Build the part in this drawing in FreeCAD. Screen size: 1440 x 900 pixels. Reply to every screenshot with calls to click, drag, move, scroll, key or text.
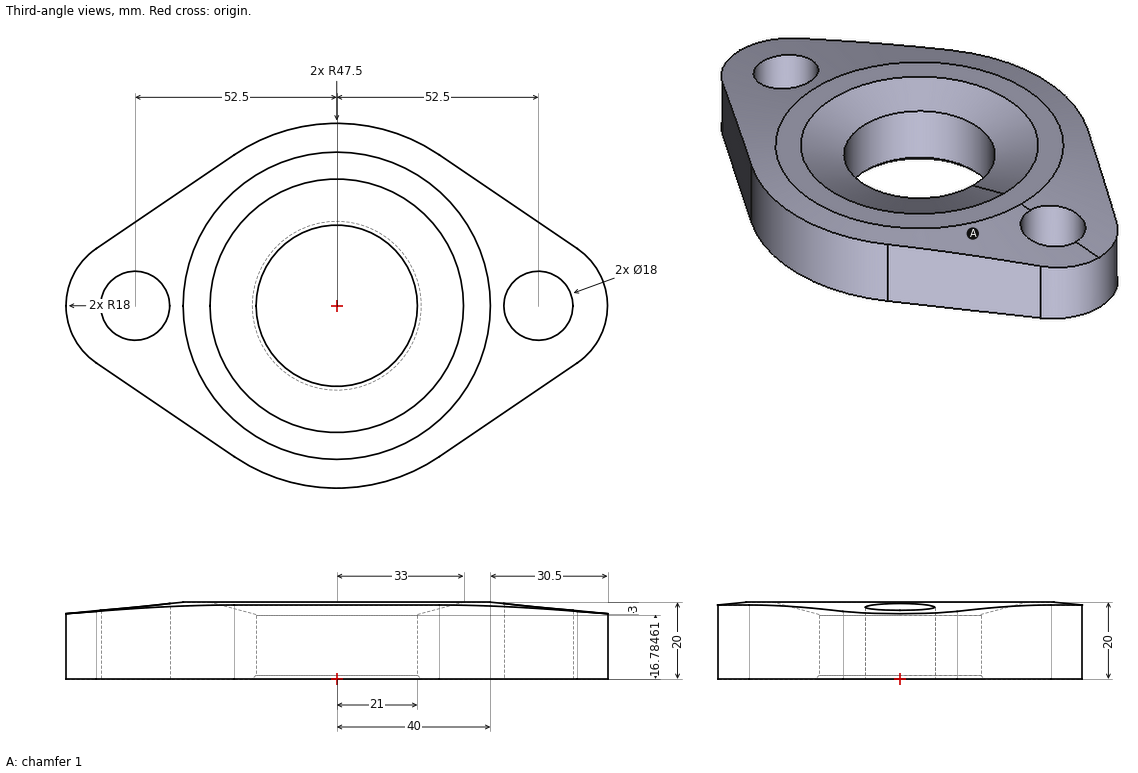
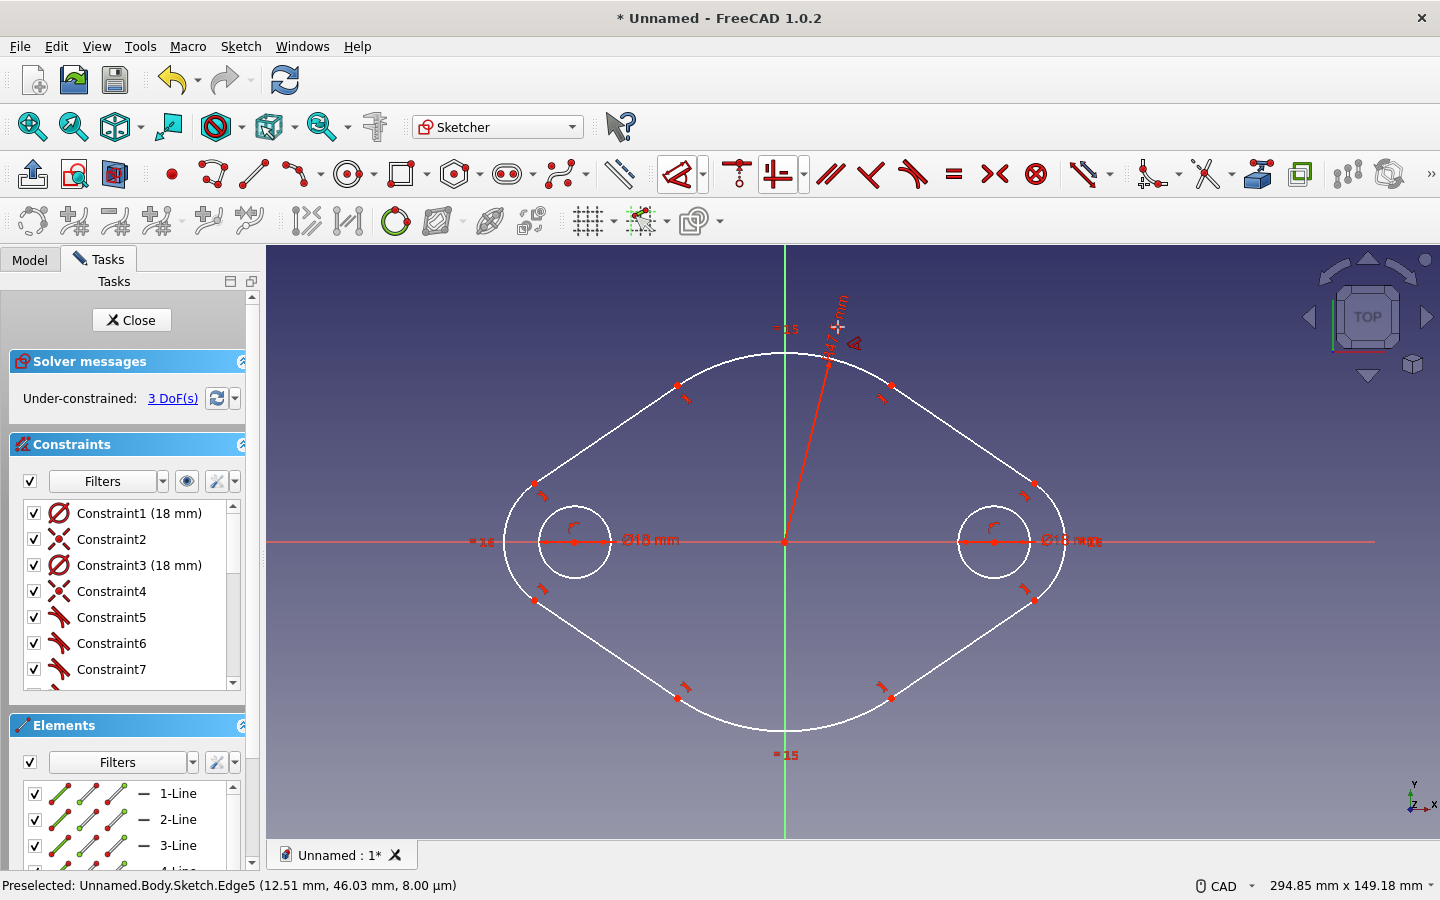
click(509, 515)
click(479, 503)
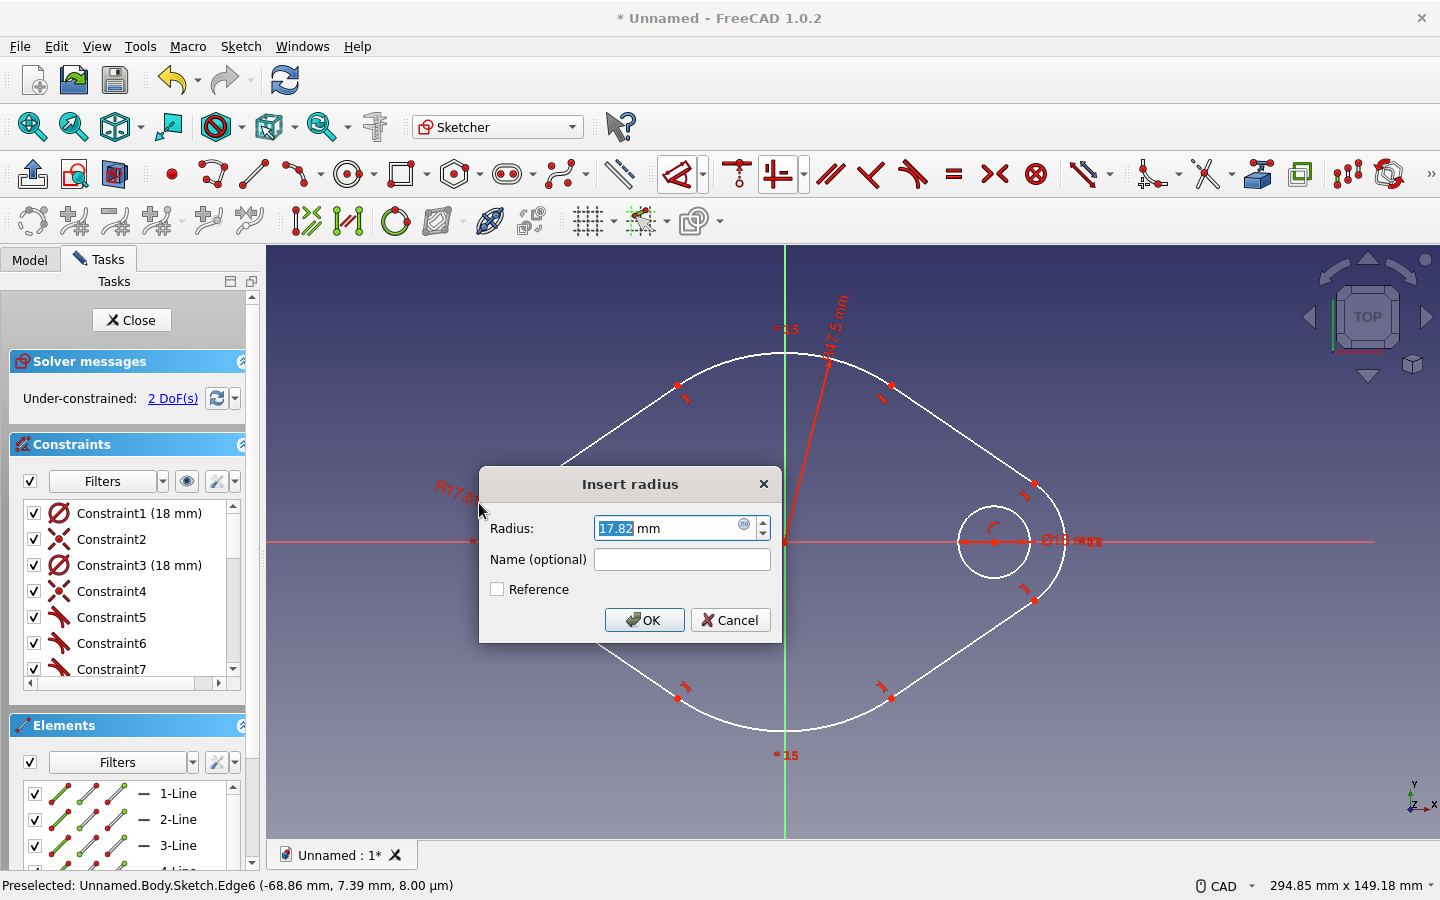
text(18)
key(Return)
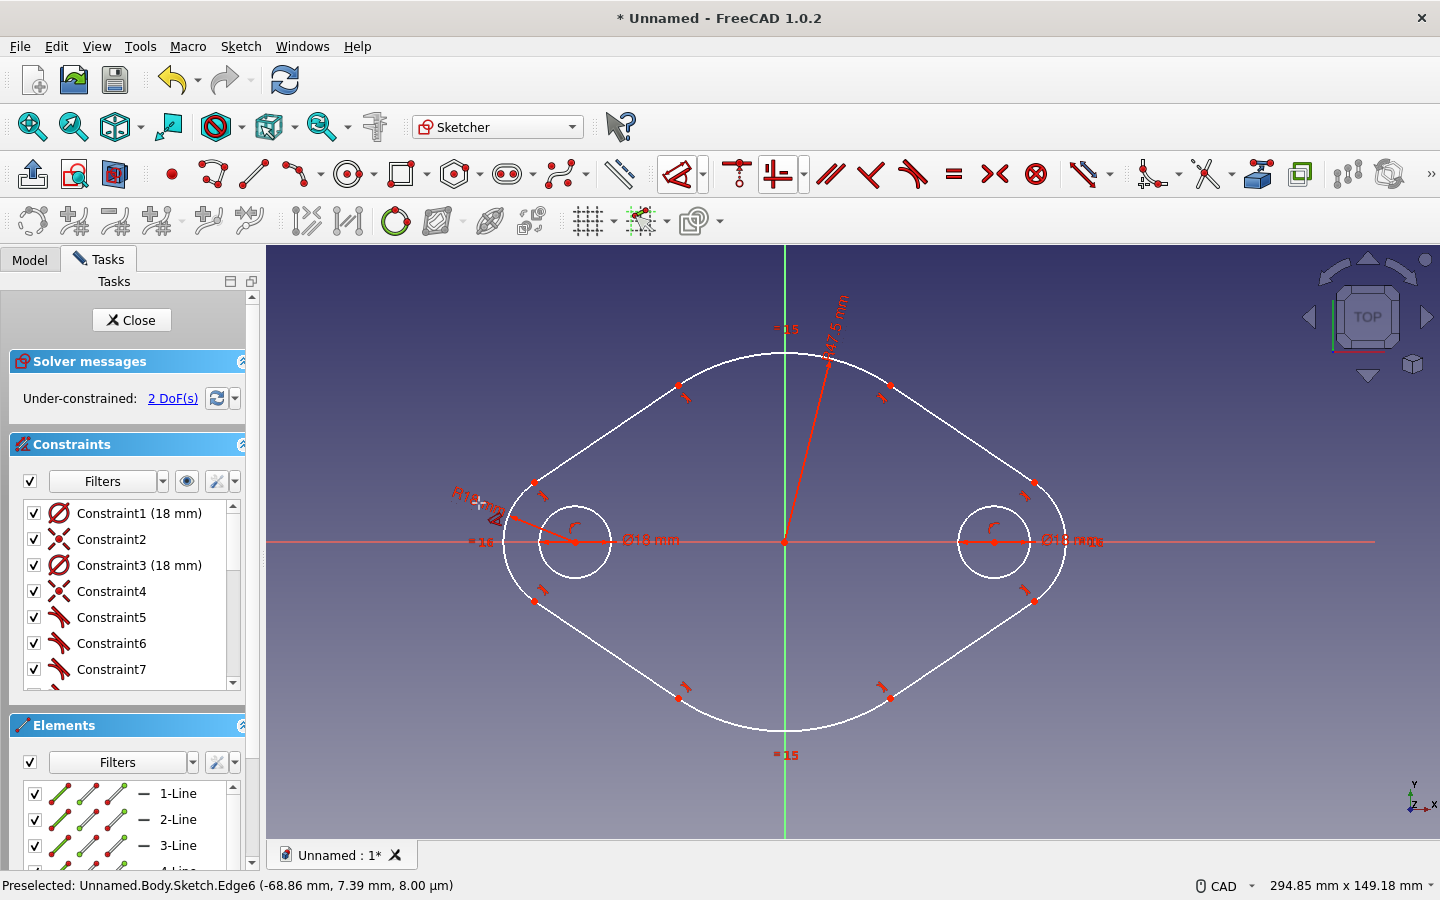
click(994, 542)
click(889, 576)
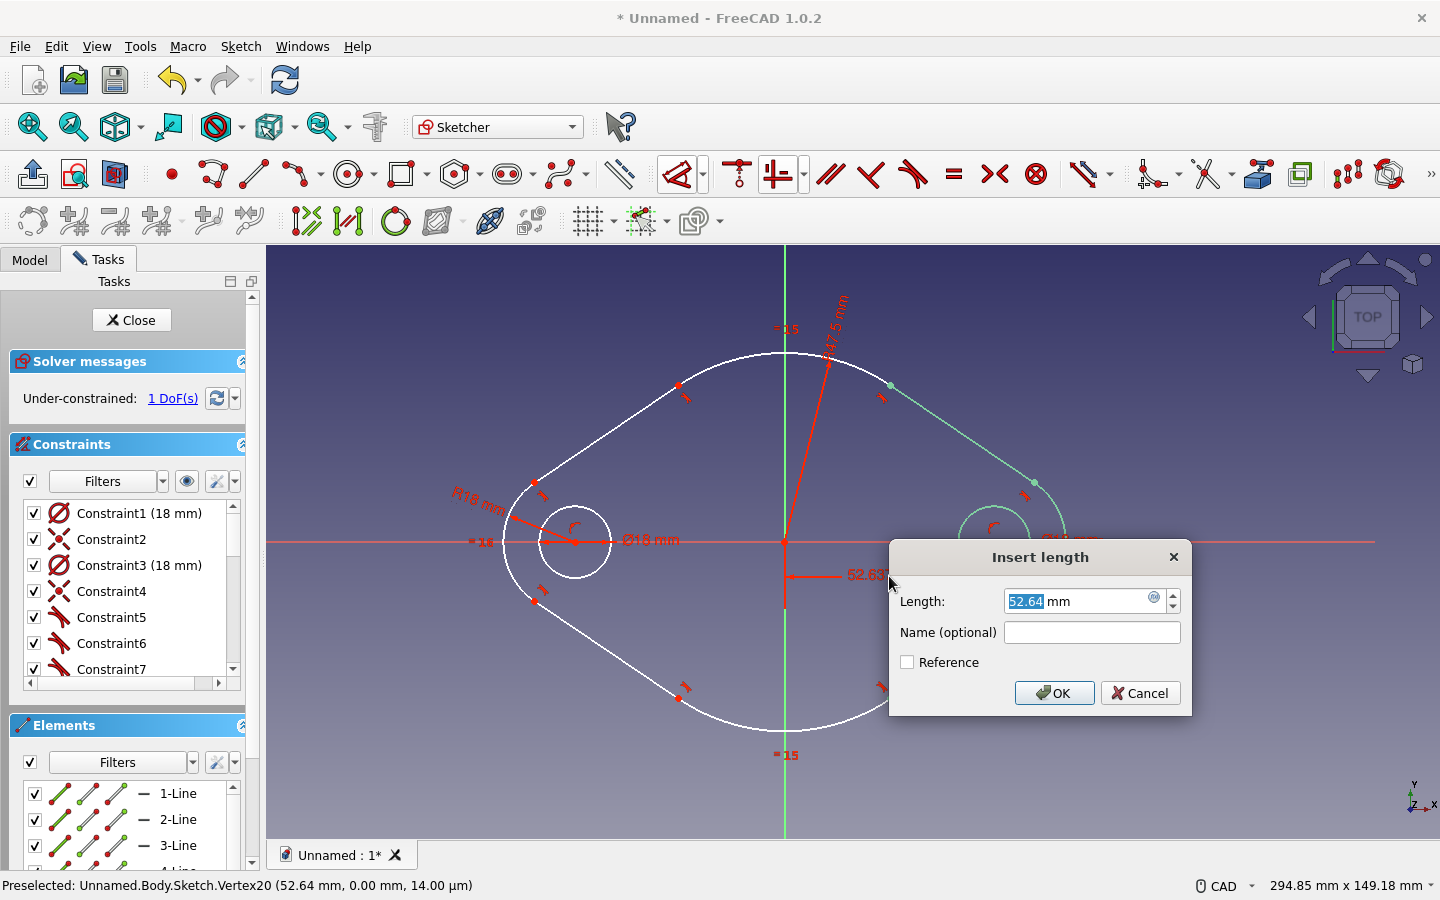
text(52.5)
key(Return)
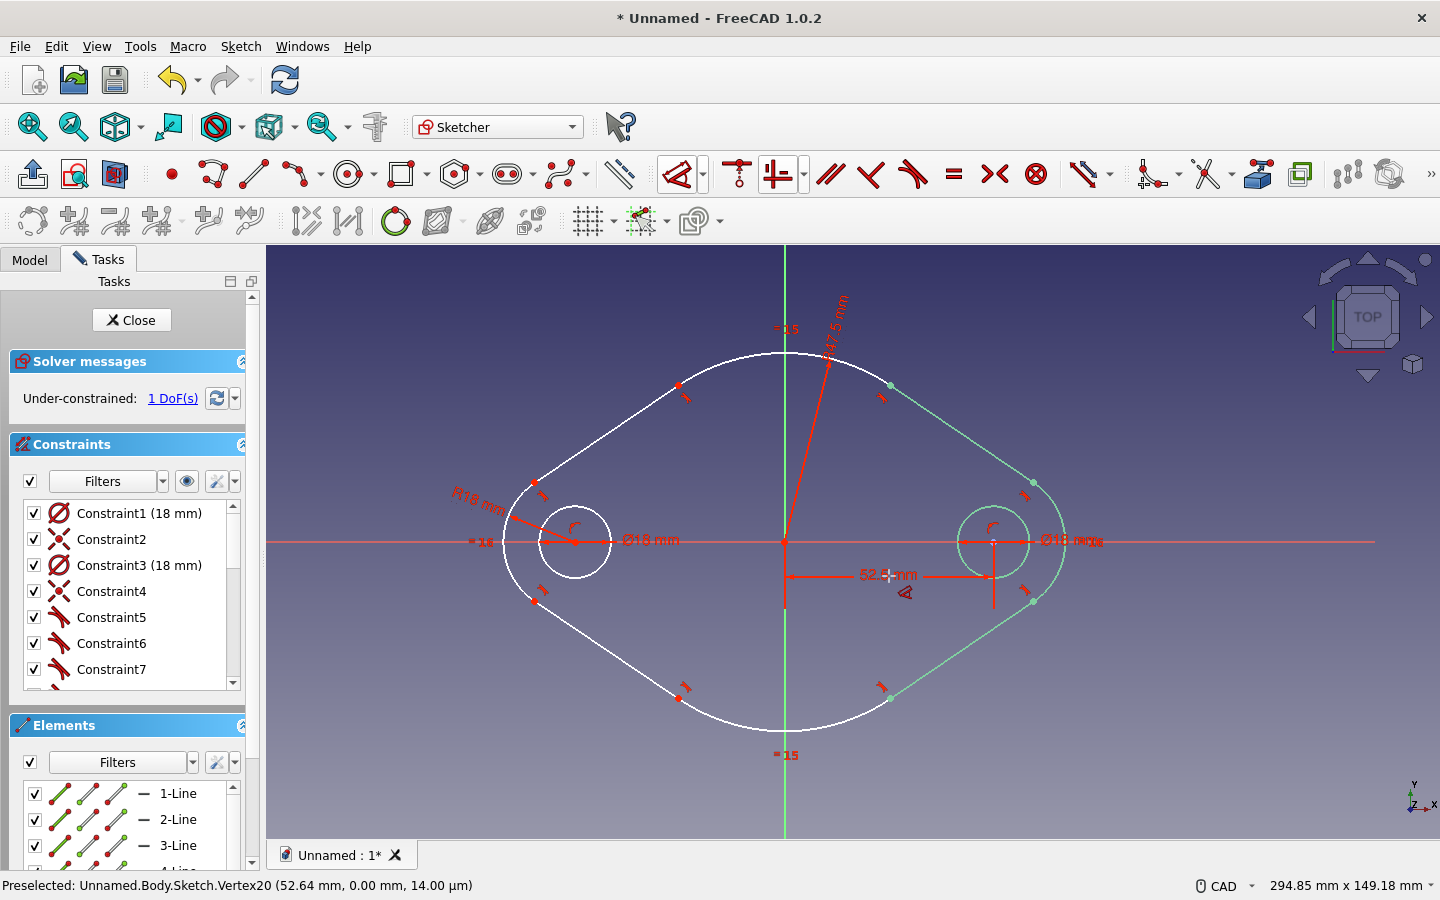
click(575, 542)
click(680, 576)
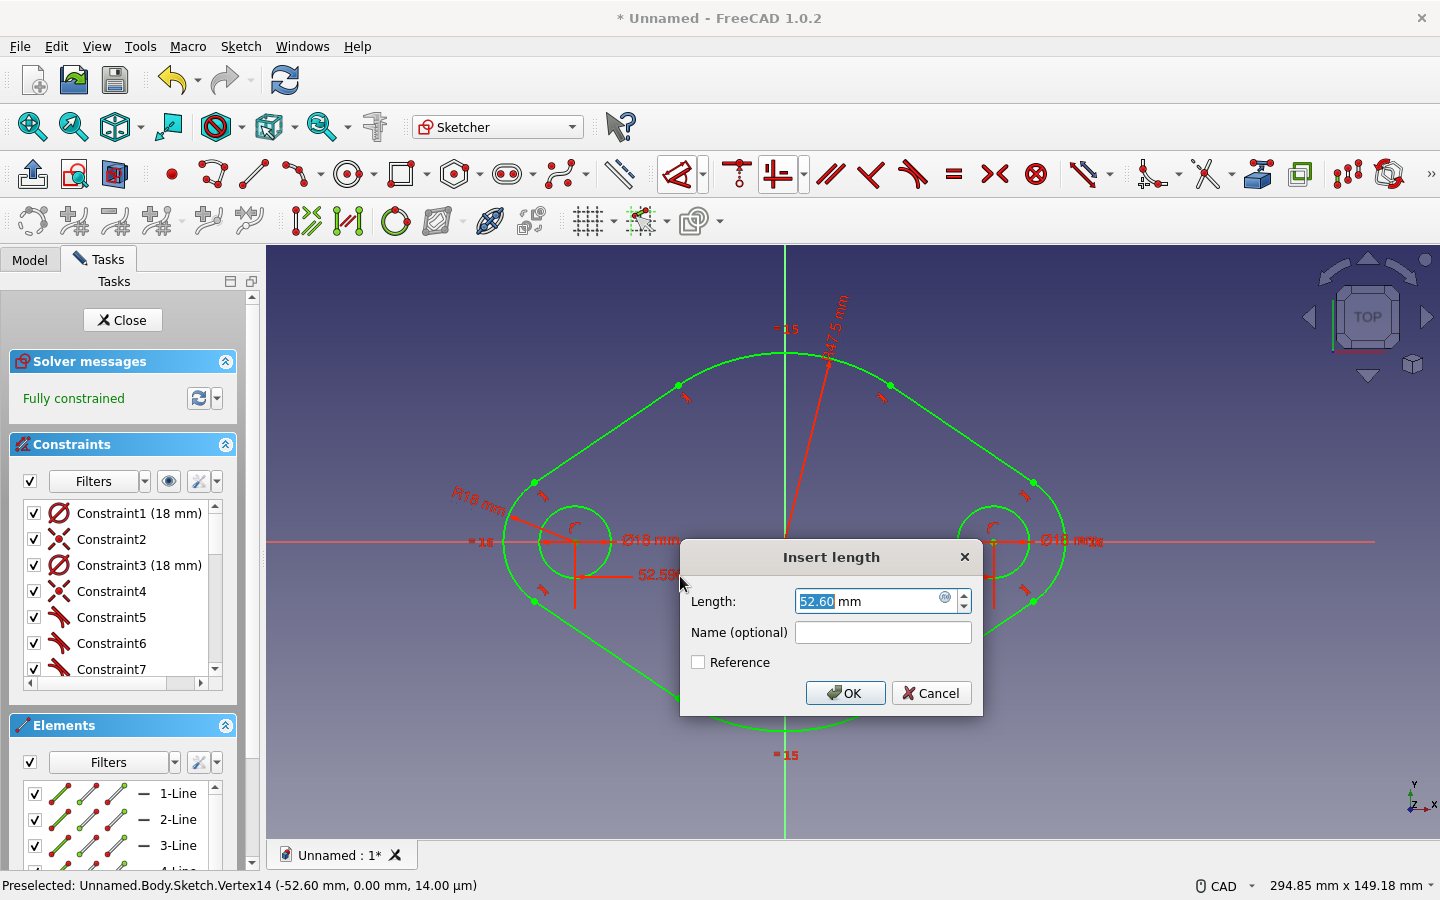
text(52.5)
key(Return)
key(Escape)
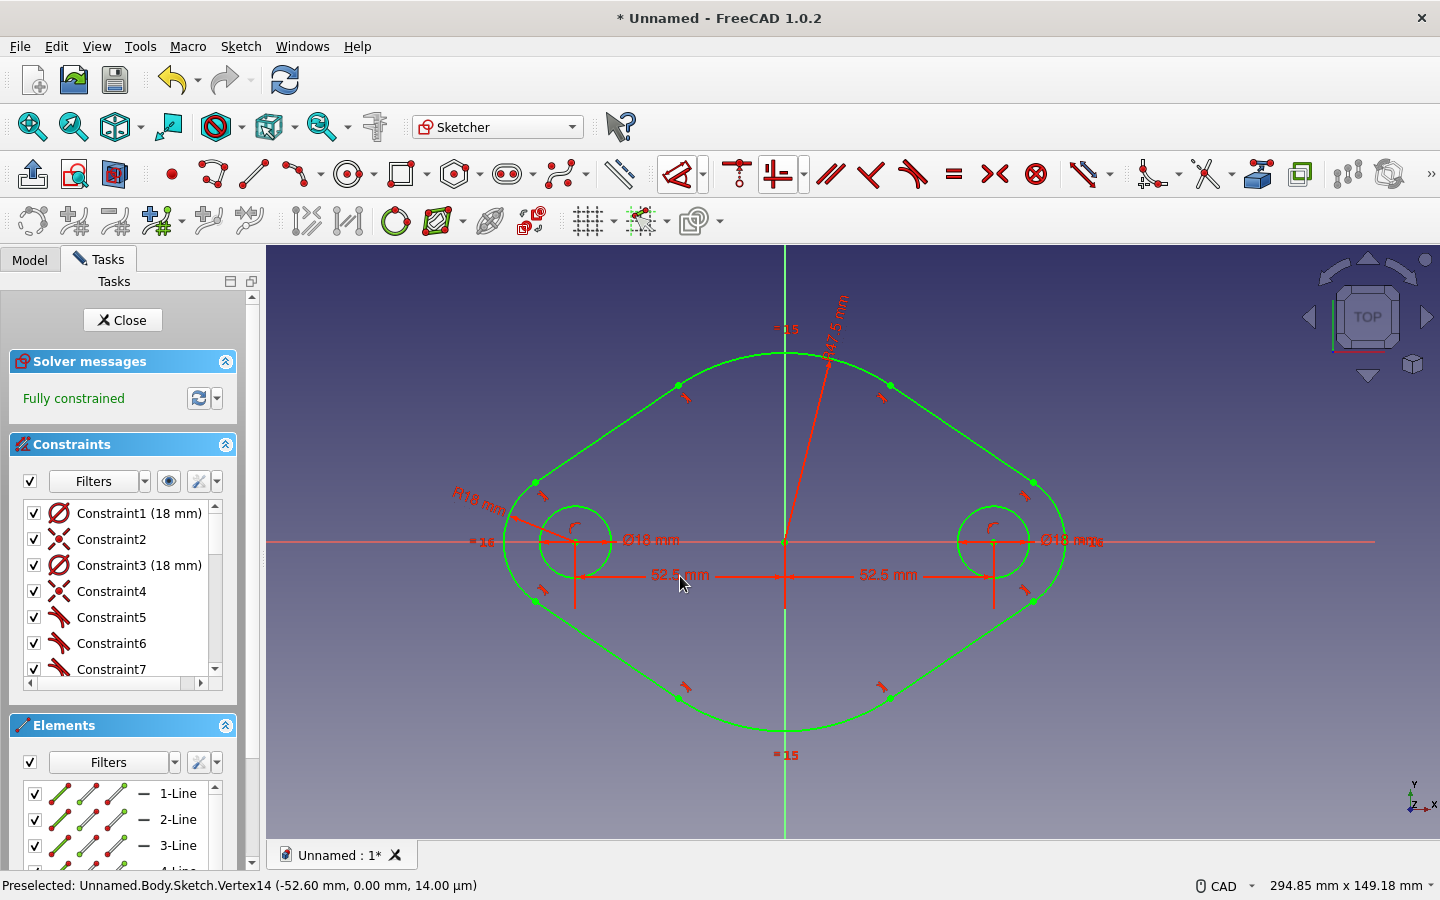
click(123, 320)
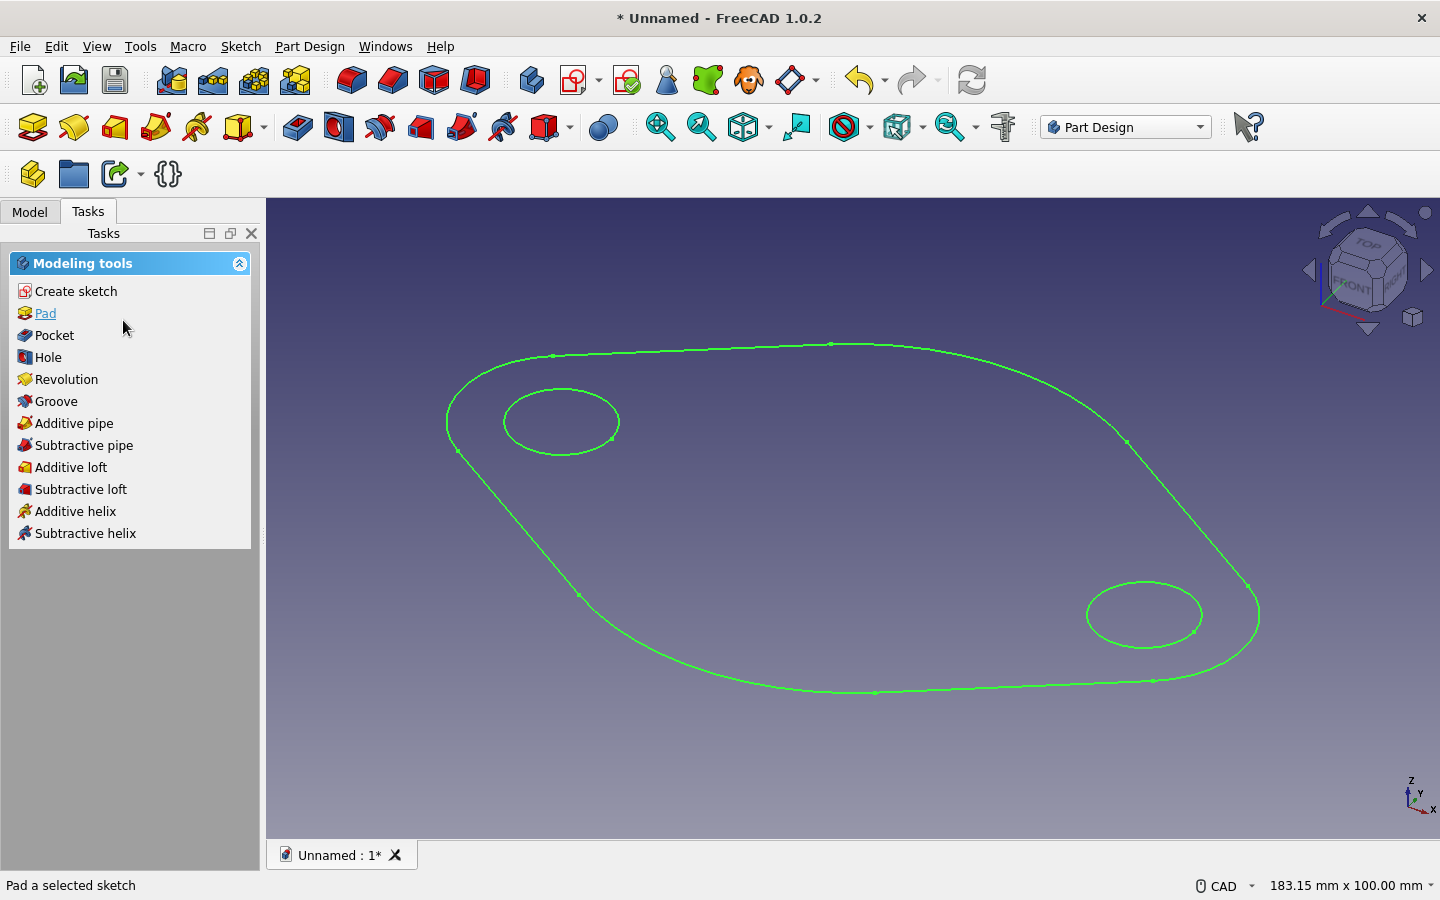
click(33, 128)